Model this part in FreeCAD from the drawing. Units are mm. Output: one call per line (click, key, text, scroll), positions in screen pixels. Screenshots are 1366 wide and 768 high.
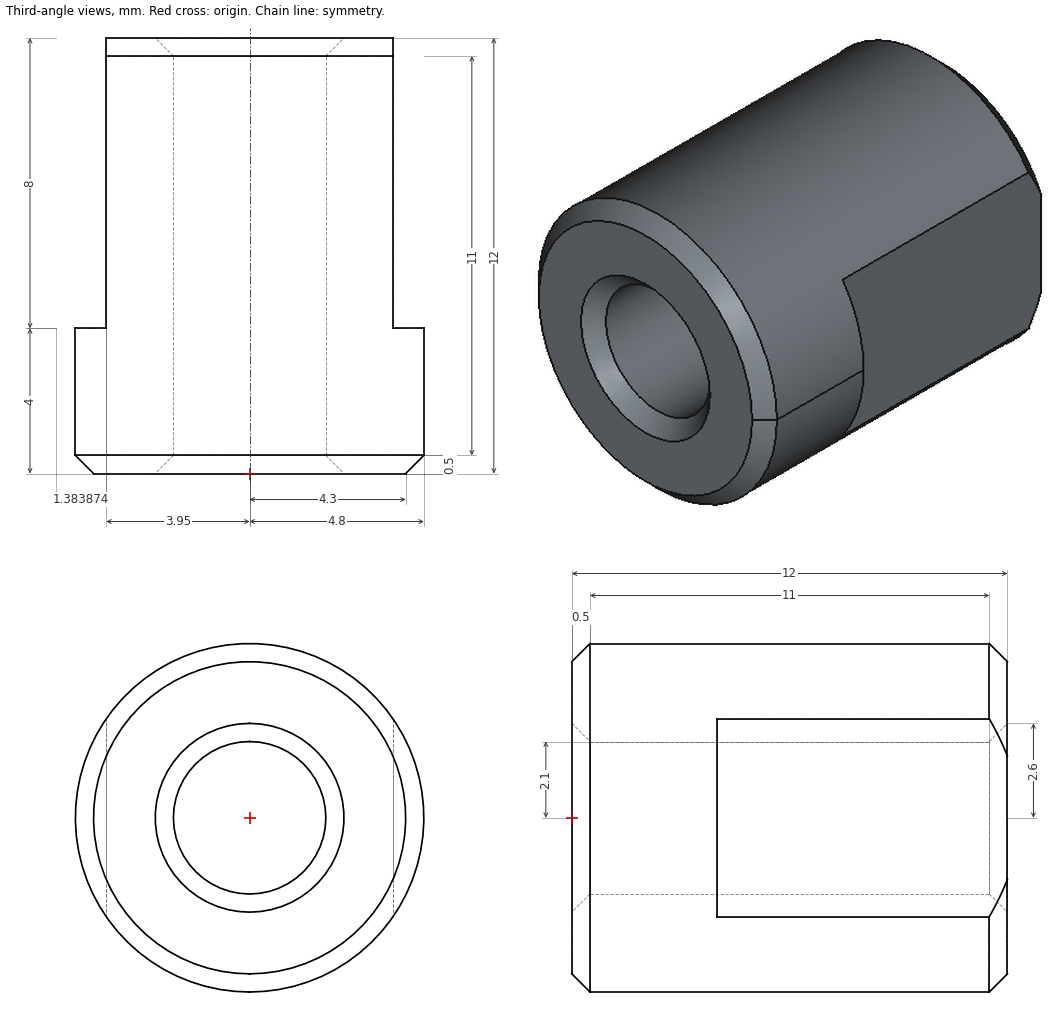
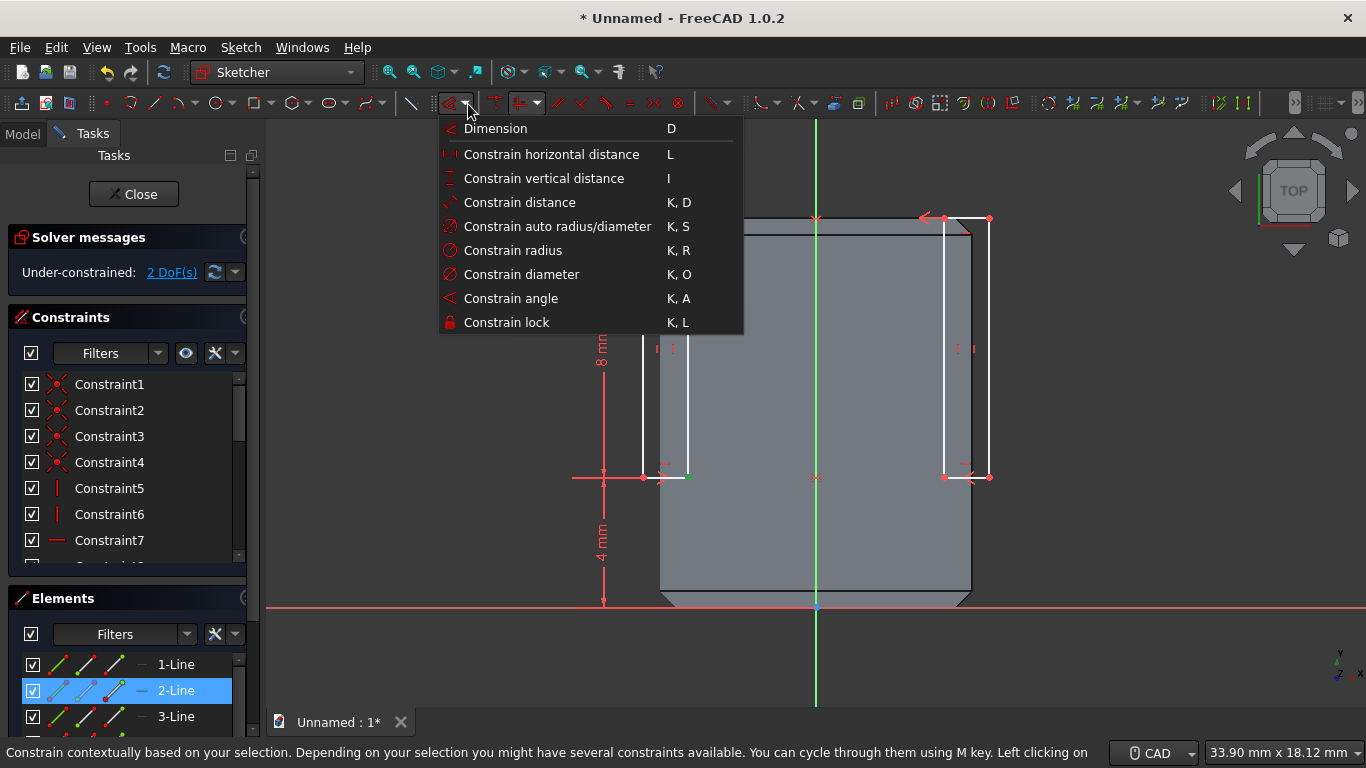
click(591, 154)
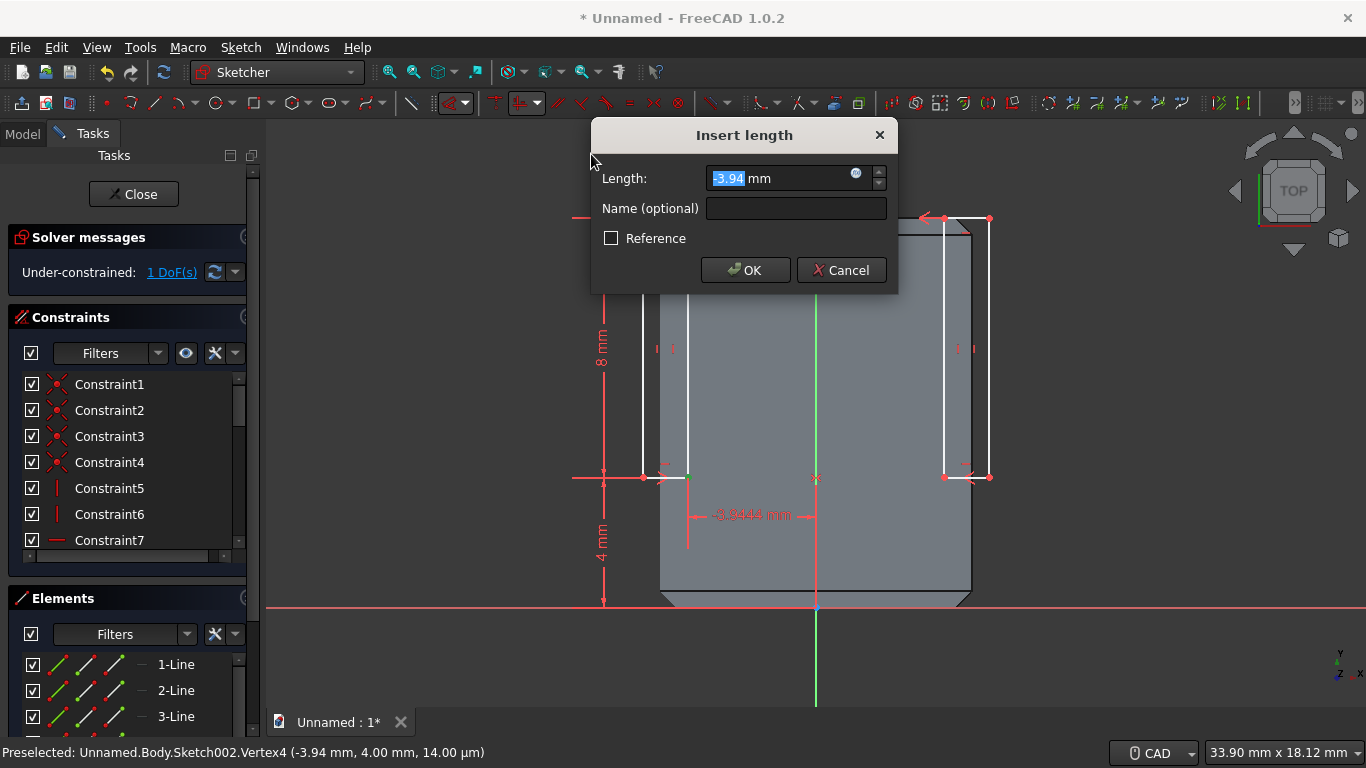
text(-3.95)
key(Return)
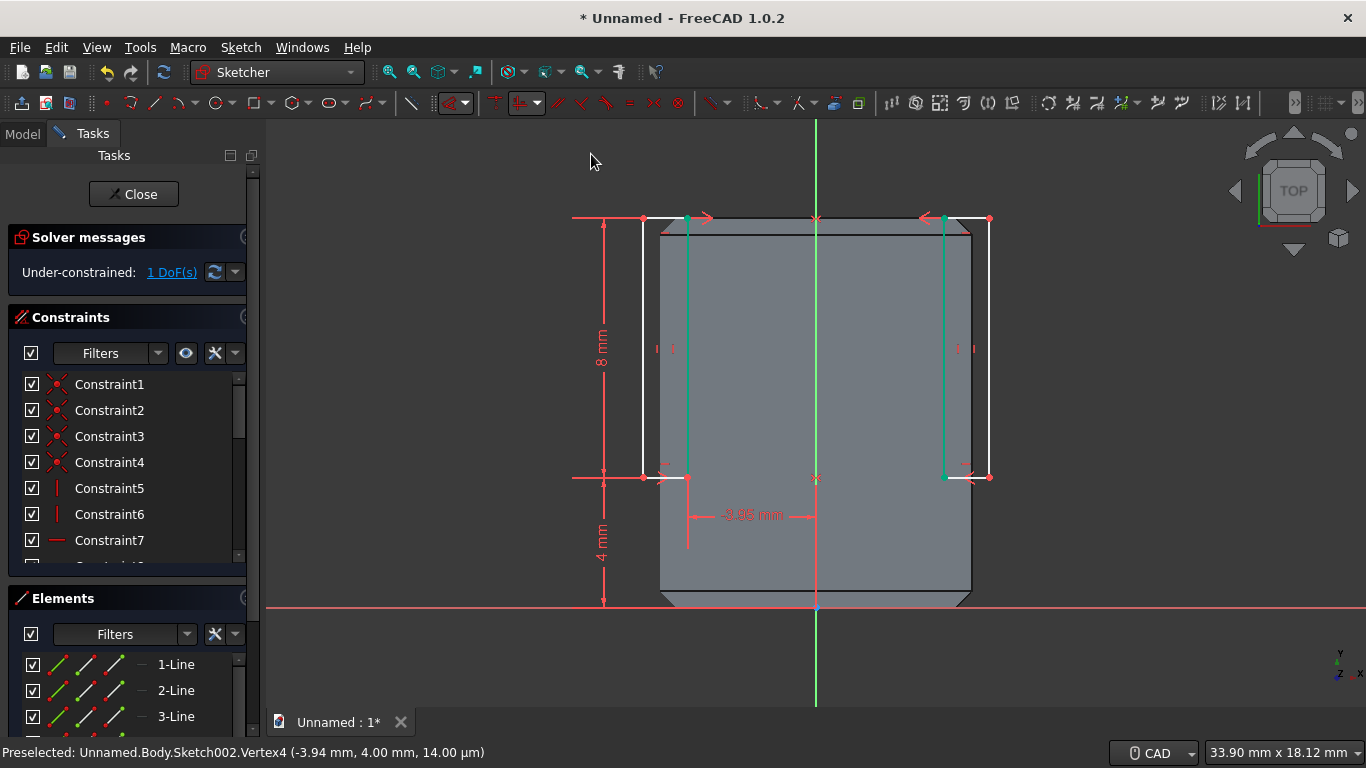
click(656, 478)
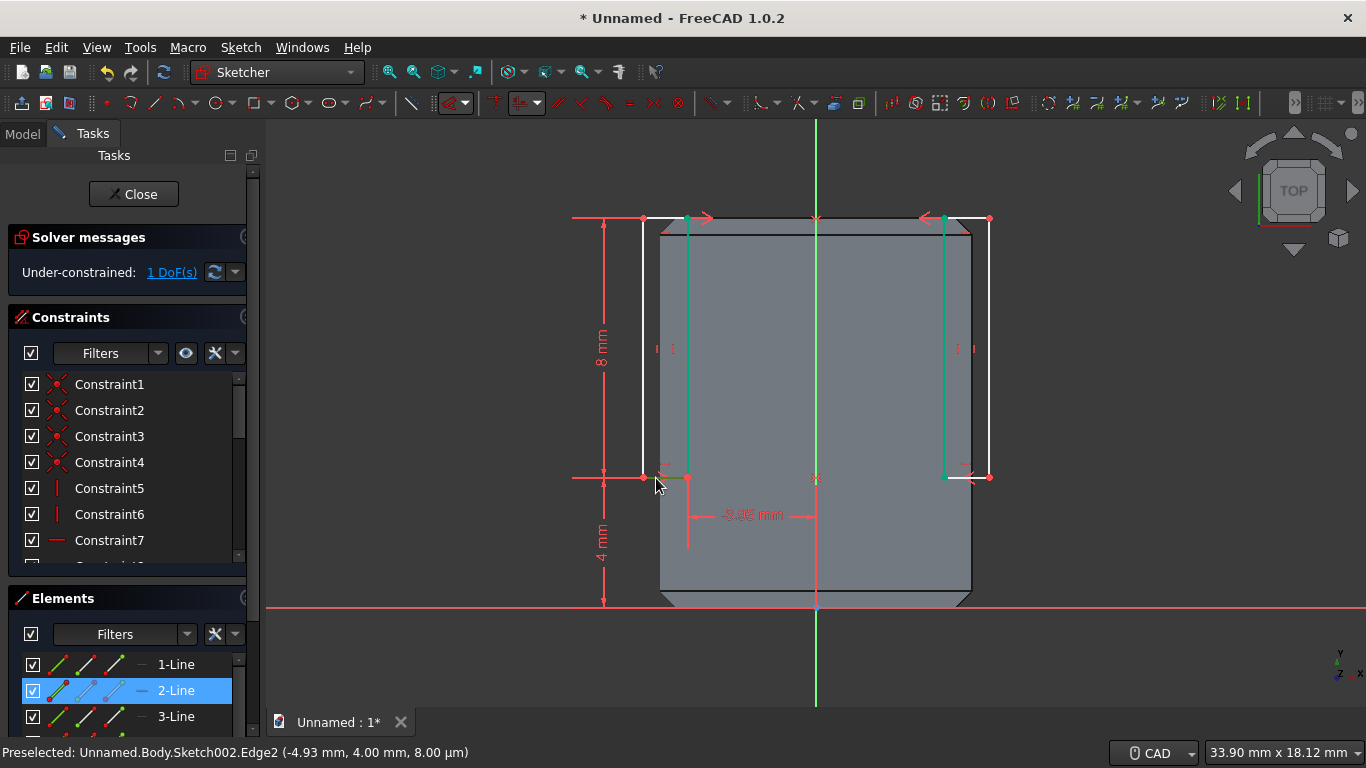
click(468, 104)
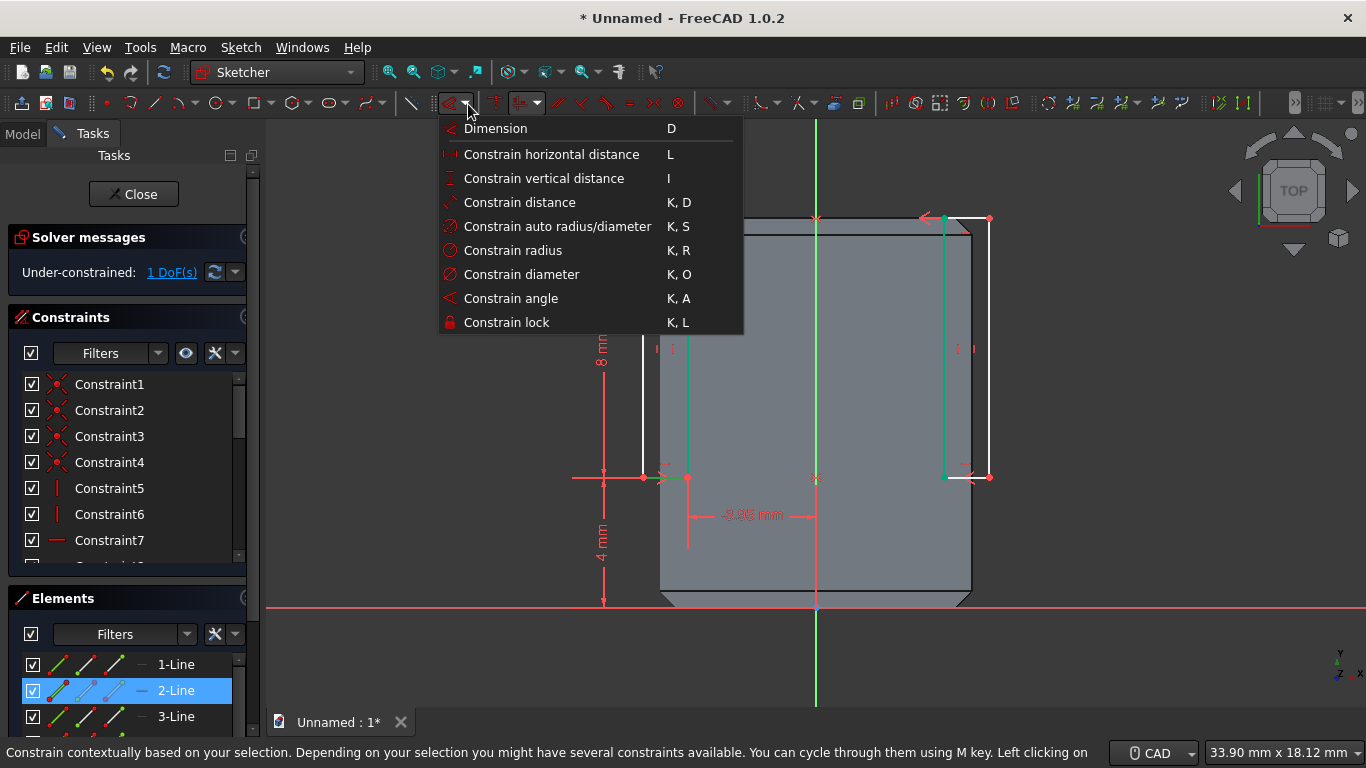
click(591, 154)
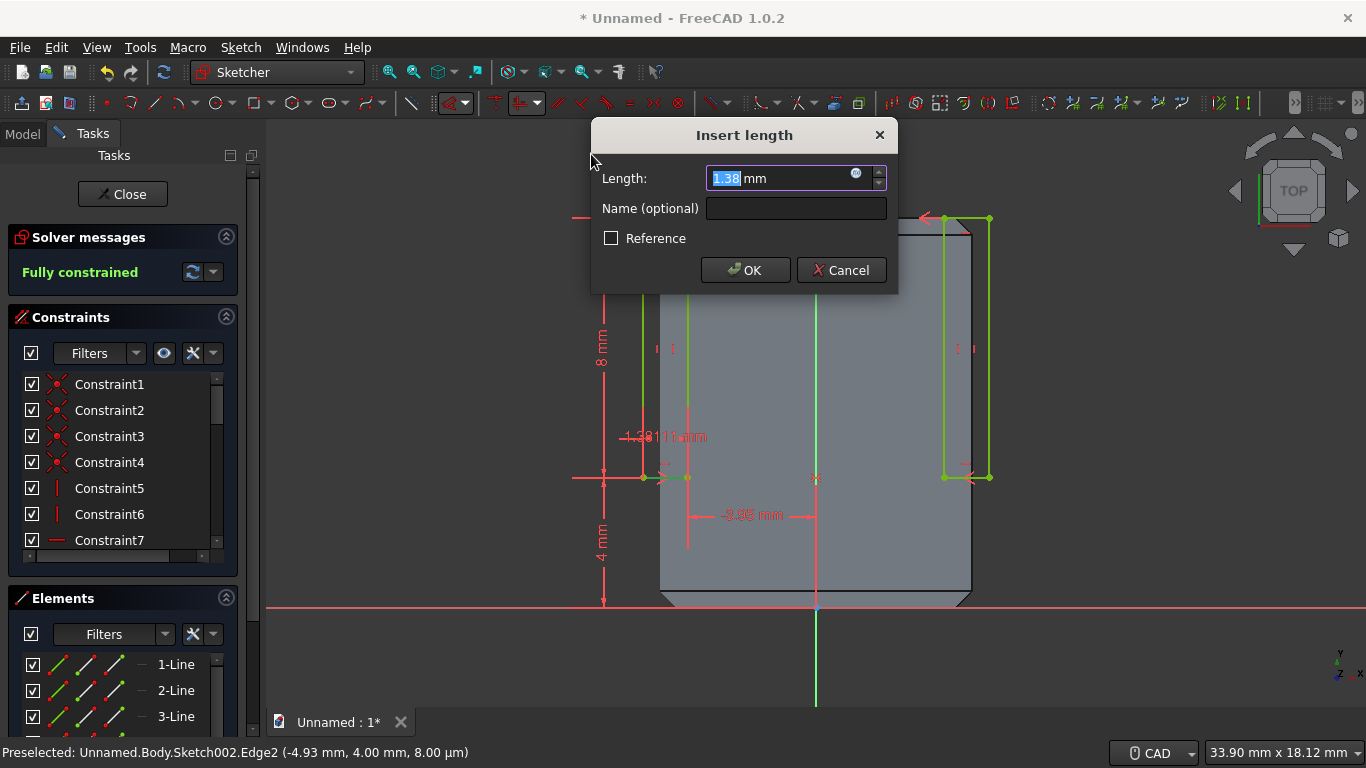
text(1.383874)
key(Return)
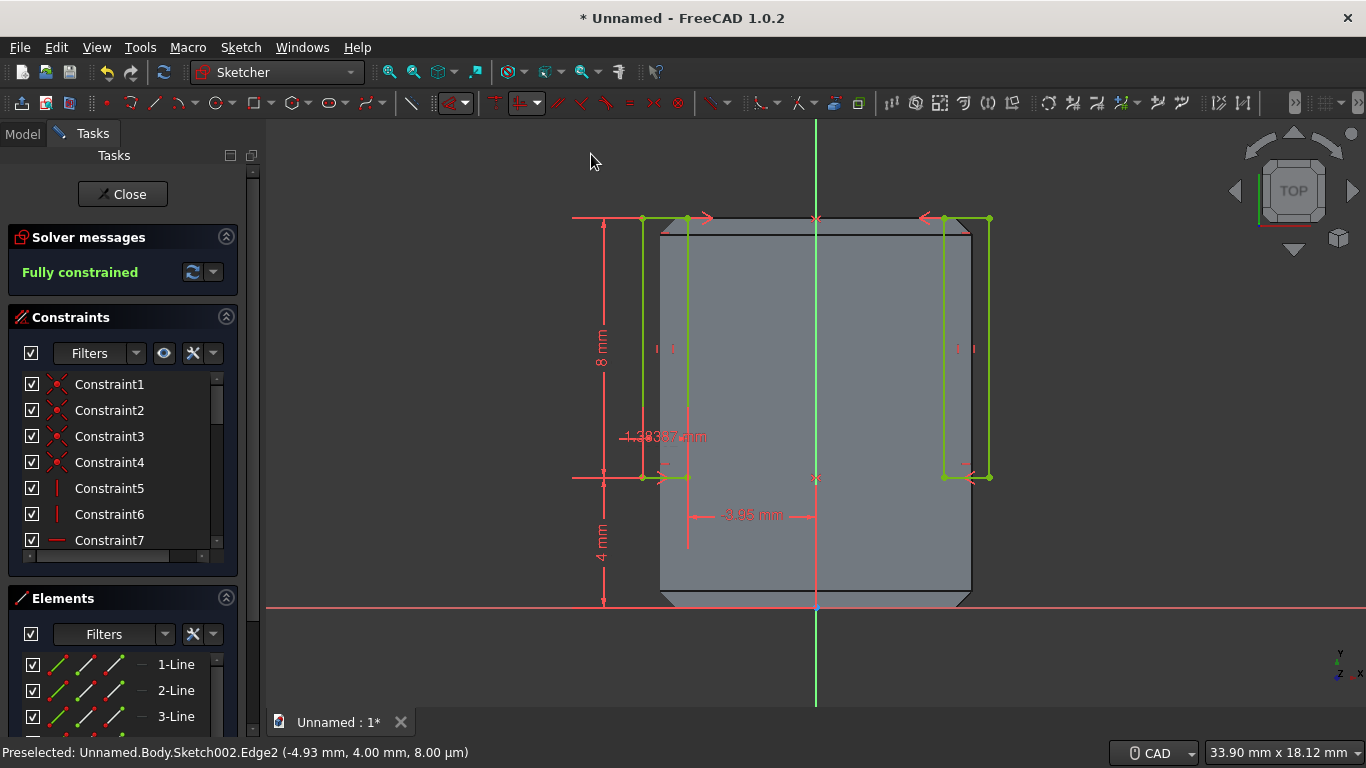
click(123, 194)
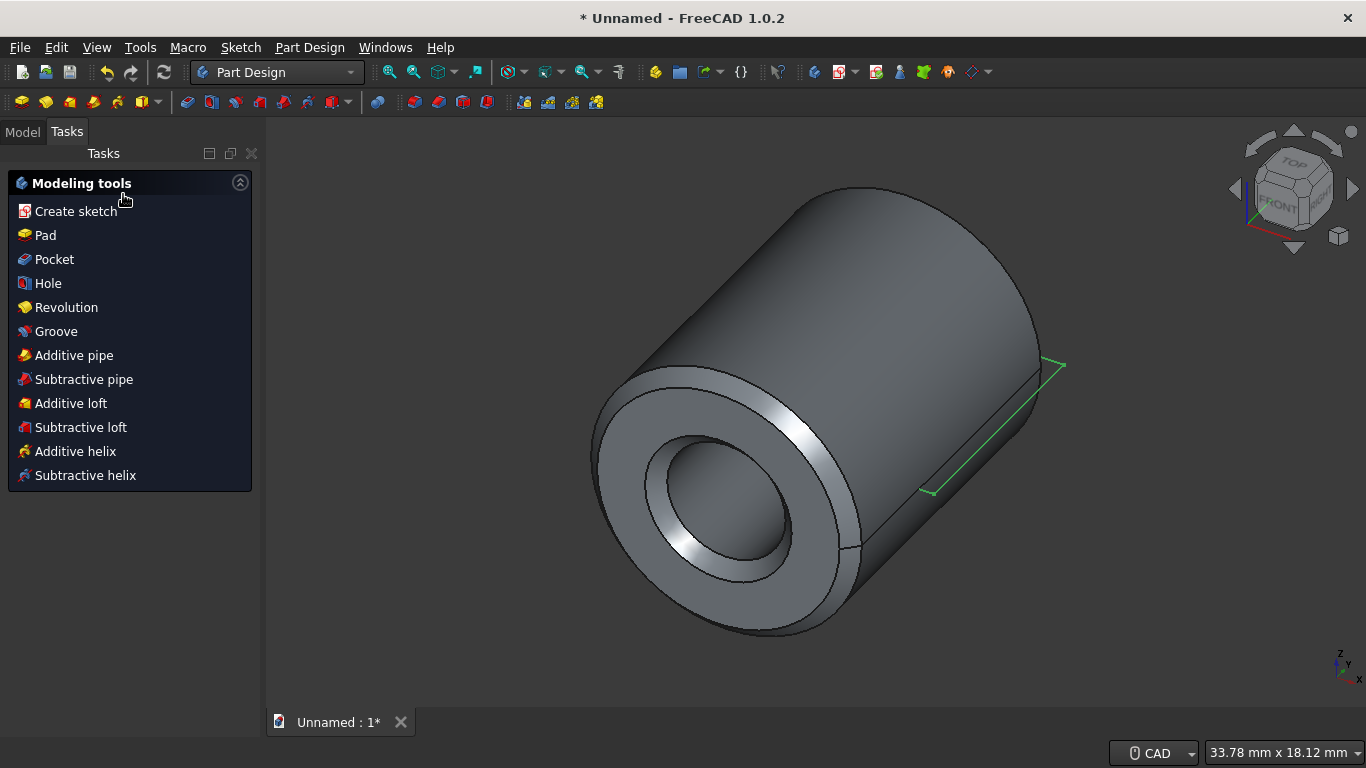
click(188, 102)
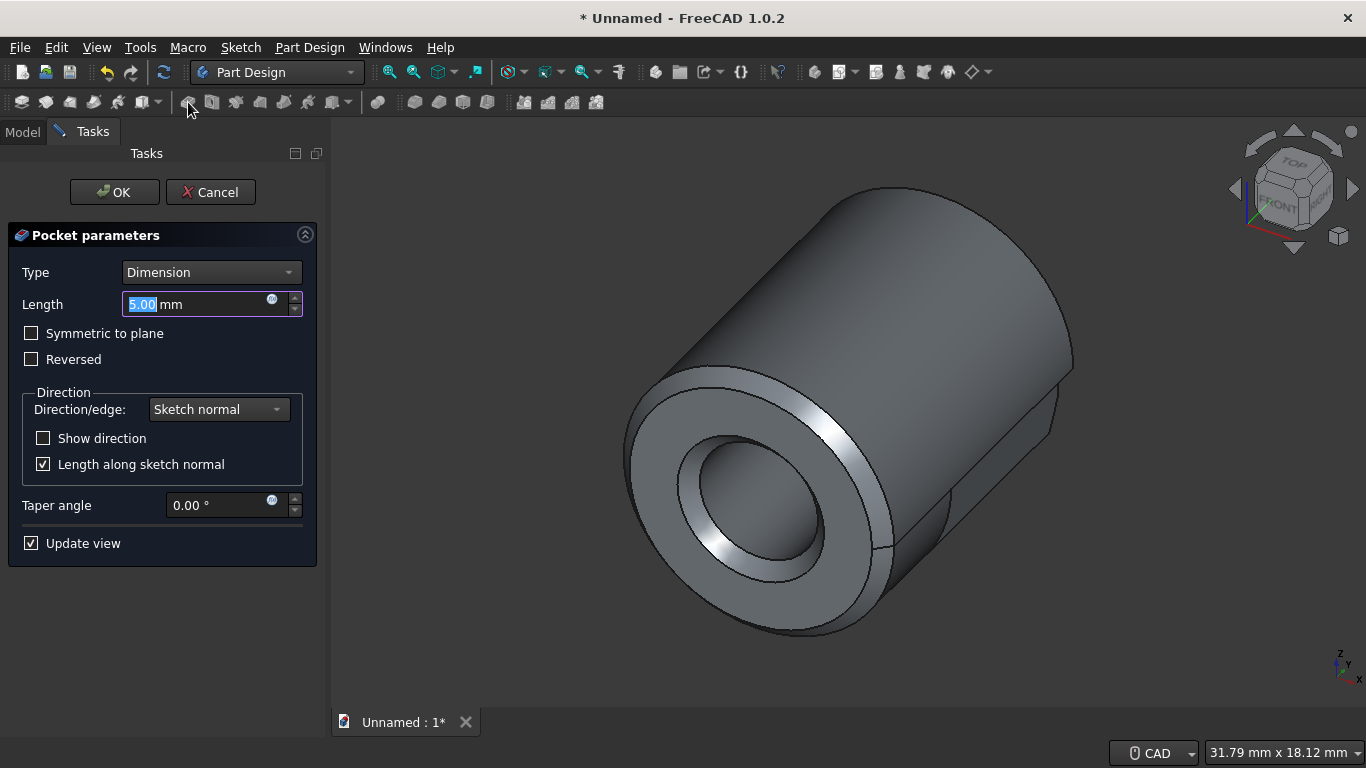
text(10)
key(Tab)